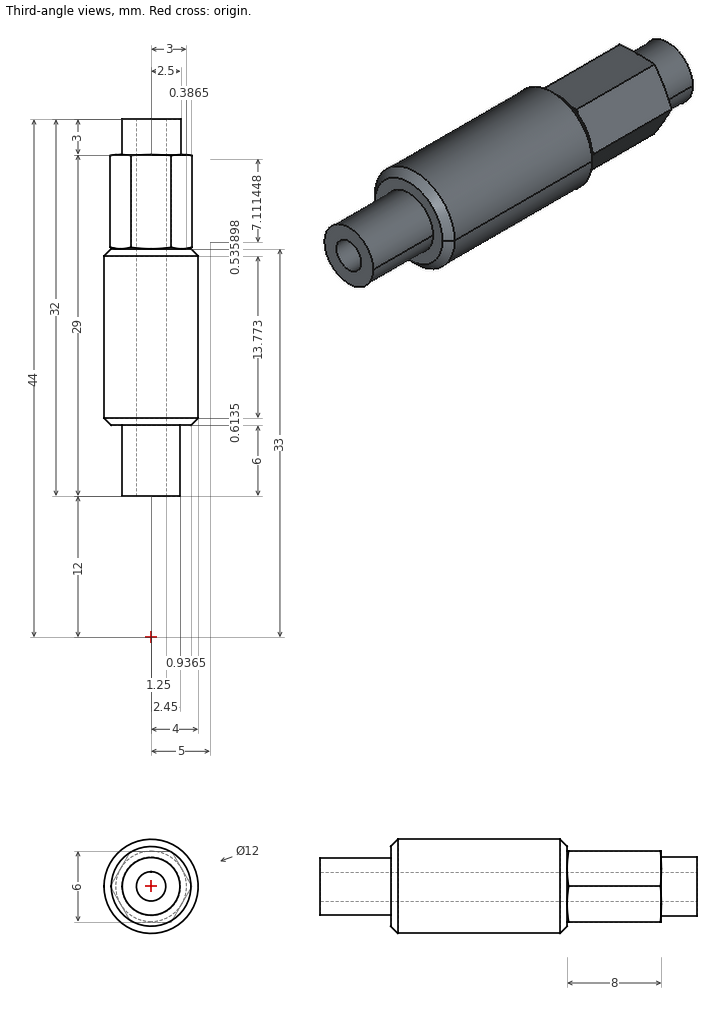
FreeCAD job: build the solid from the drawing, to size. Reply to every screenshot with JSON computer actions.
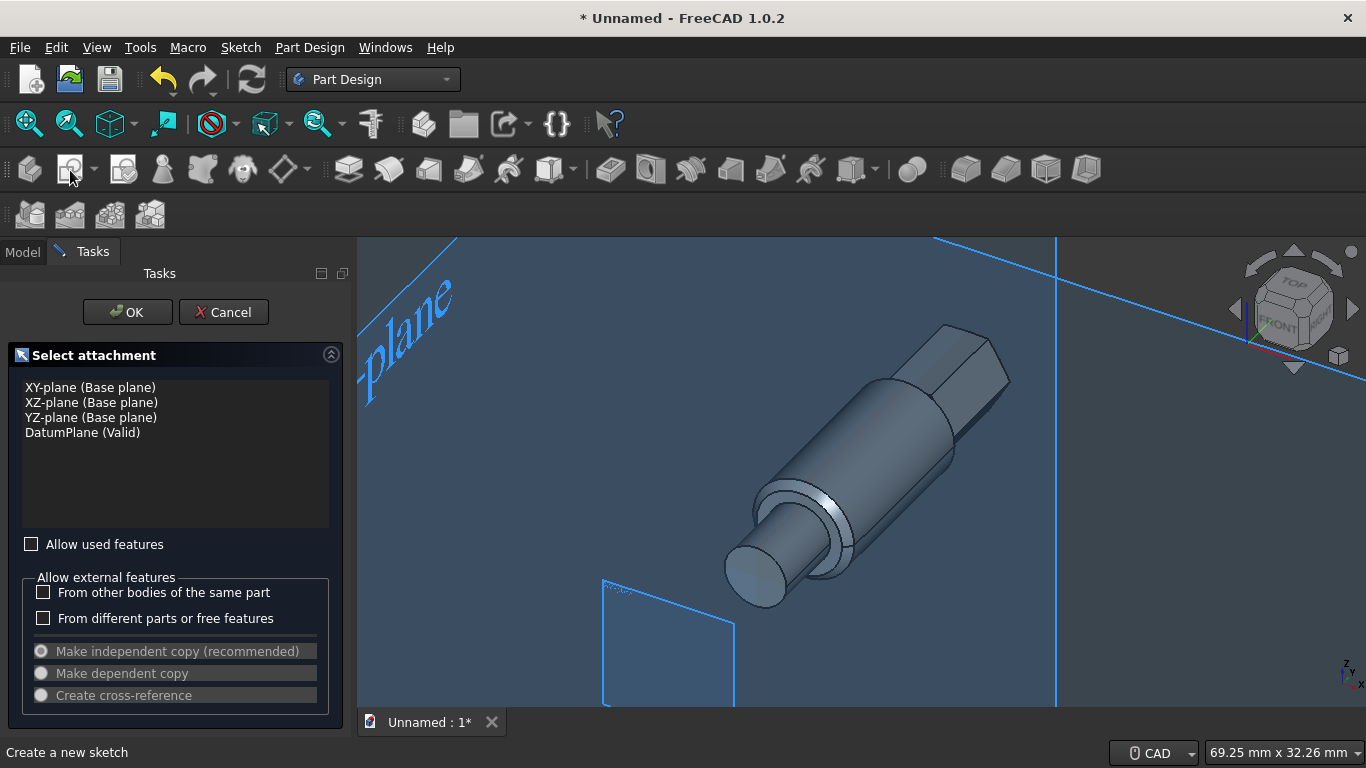
{"action": "left_click", "coordinate": [82, 388]}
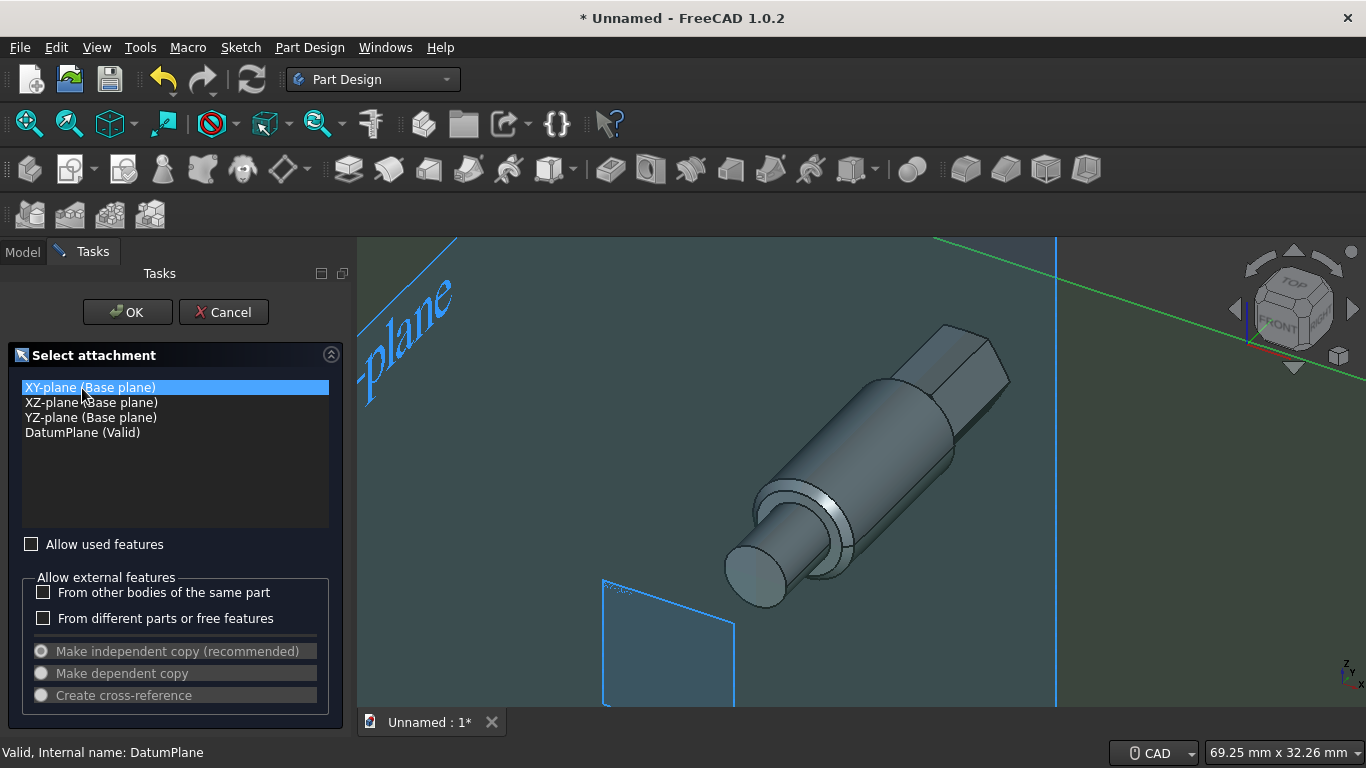
{"action": "left_click", "coordinate": [128, 312]}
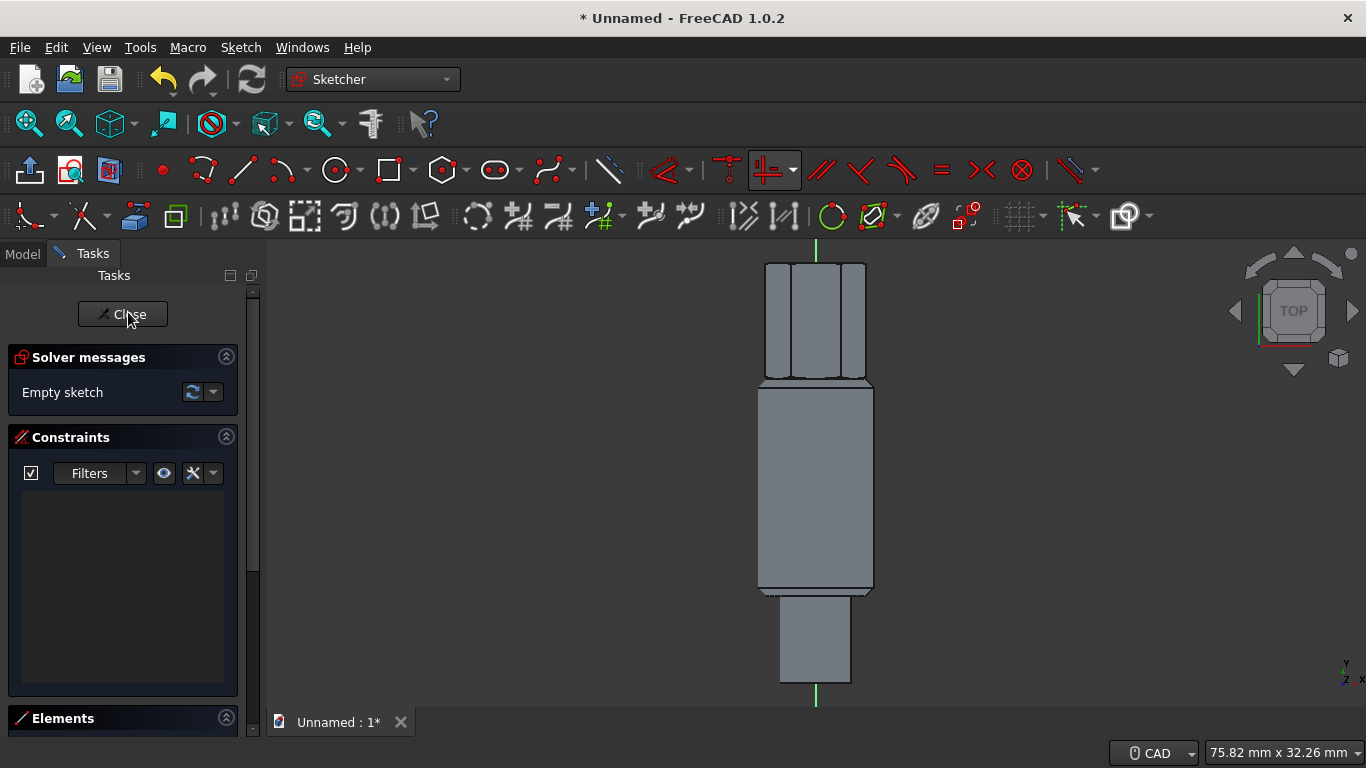
{"action": "left_click", "coordinate": [110, 170]}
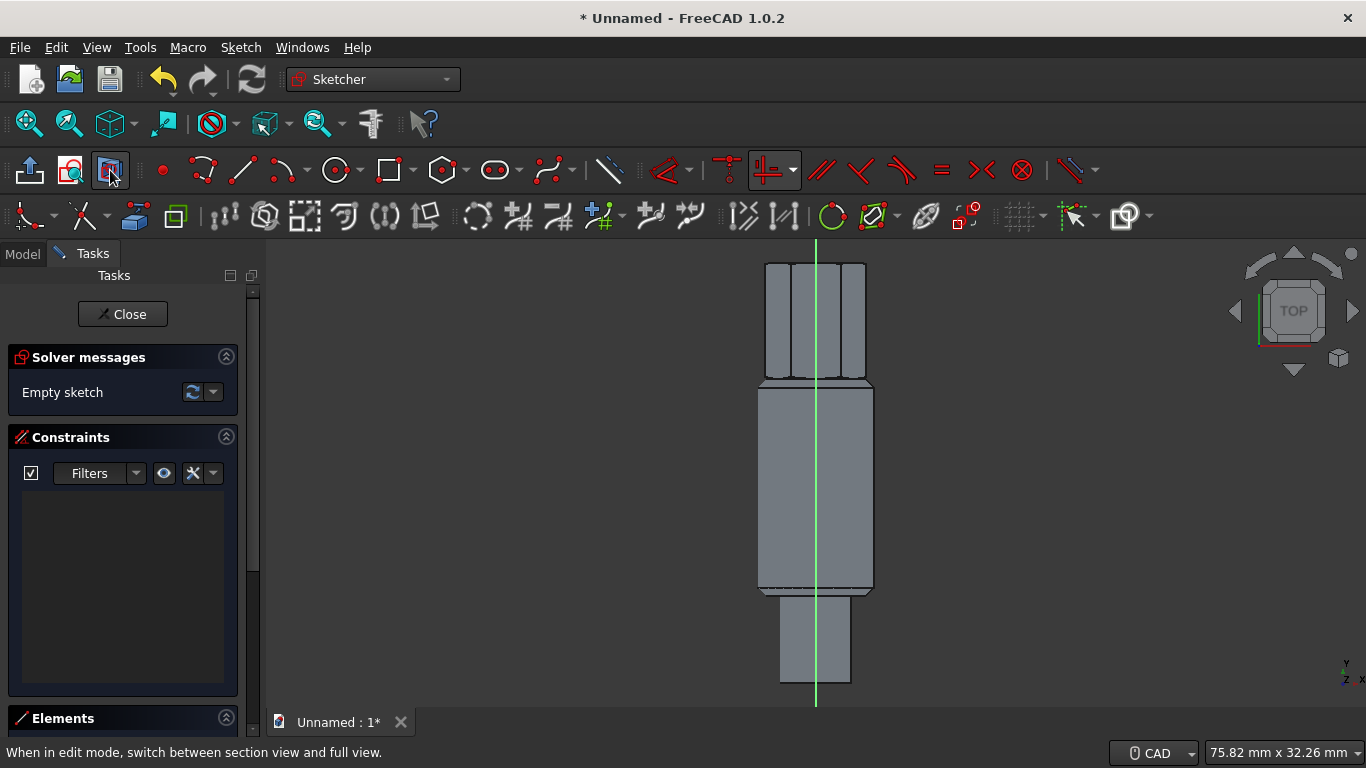
{"action": "scroll", "coordinate": [748, 473], "scroll_direction": "down", "scroll_amount": 5}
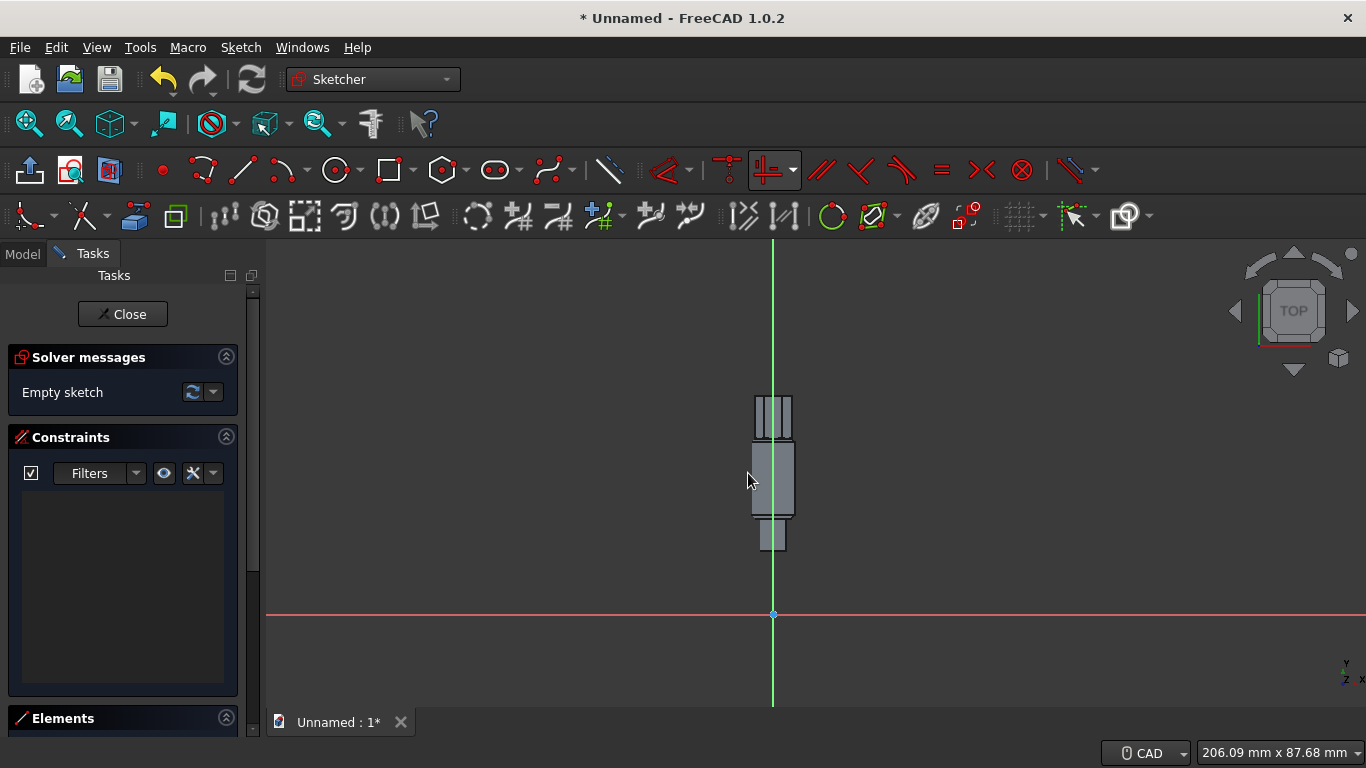
{"action": "scroll", "coordinate": [782, 382], "scroll_direction": "up", "scroll_amount": 14}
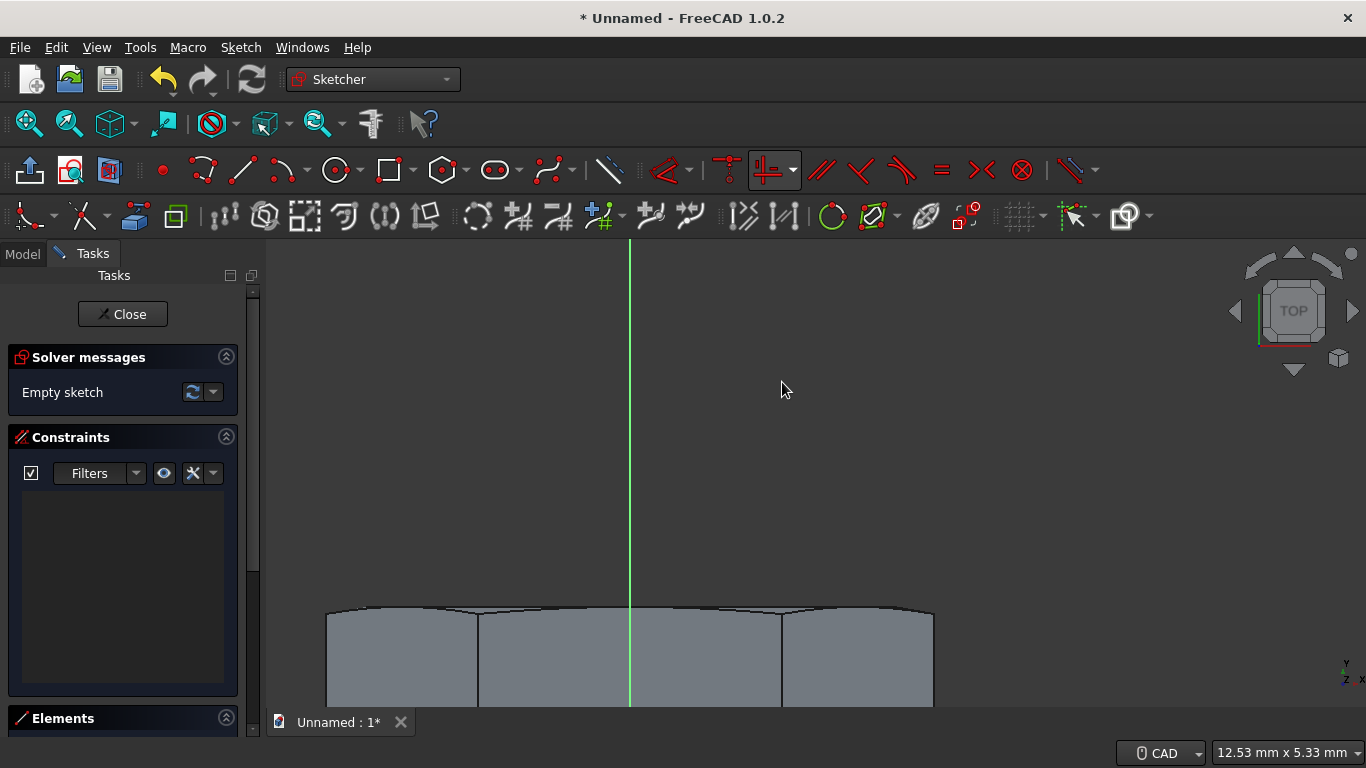
{"action": "left_click", "coordinate": [390, 170]}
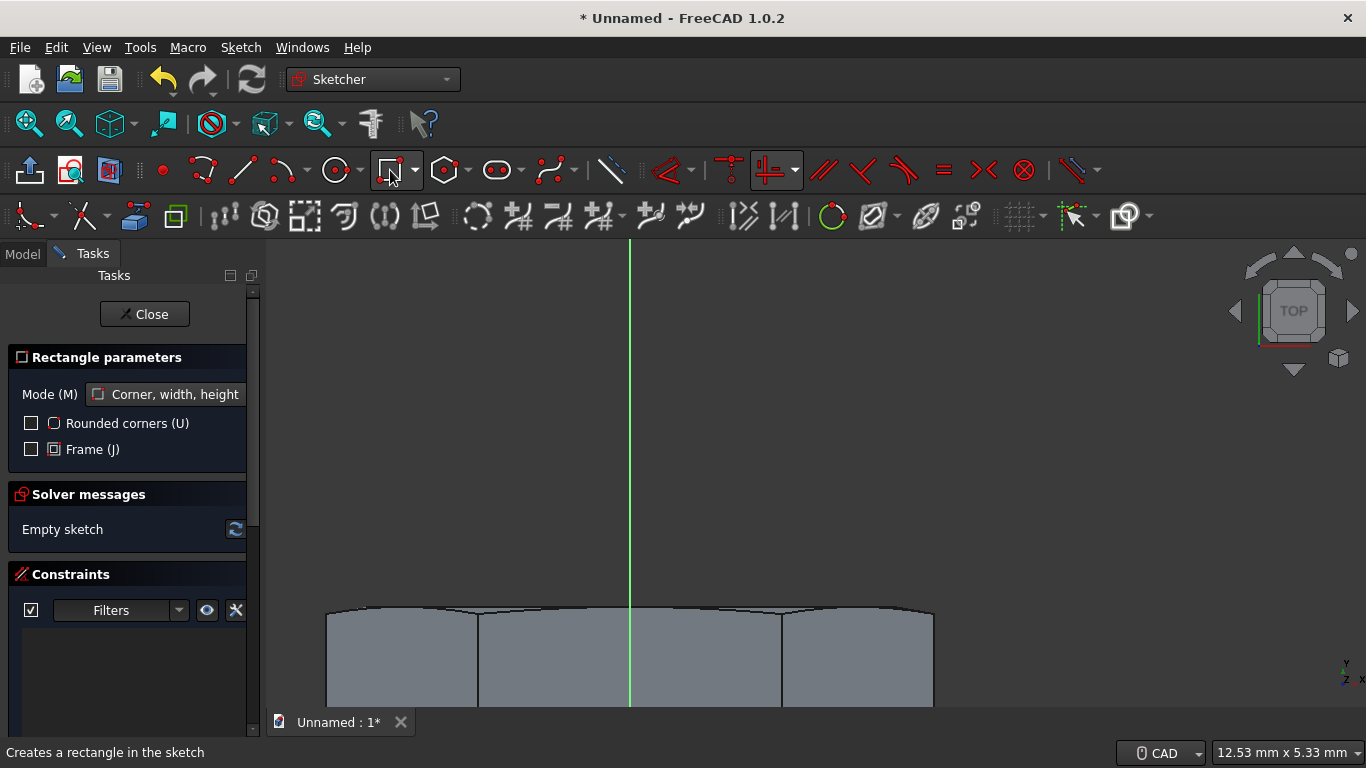
{"action": "left_click", "coordinate": [630, 344]}
{"action": "left_click", "coordinate": [849, 607]}
{"action": "key", "text": "Escape"}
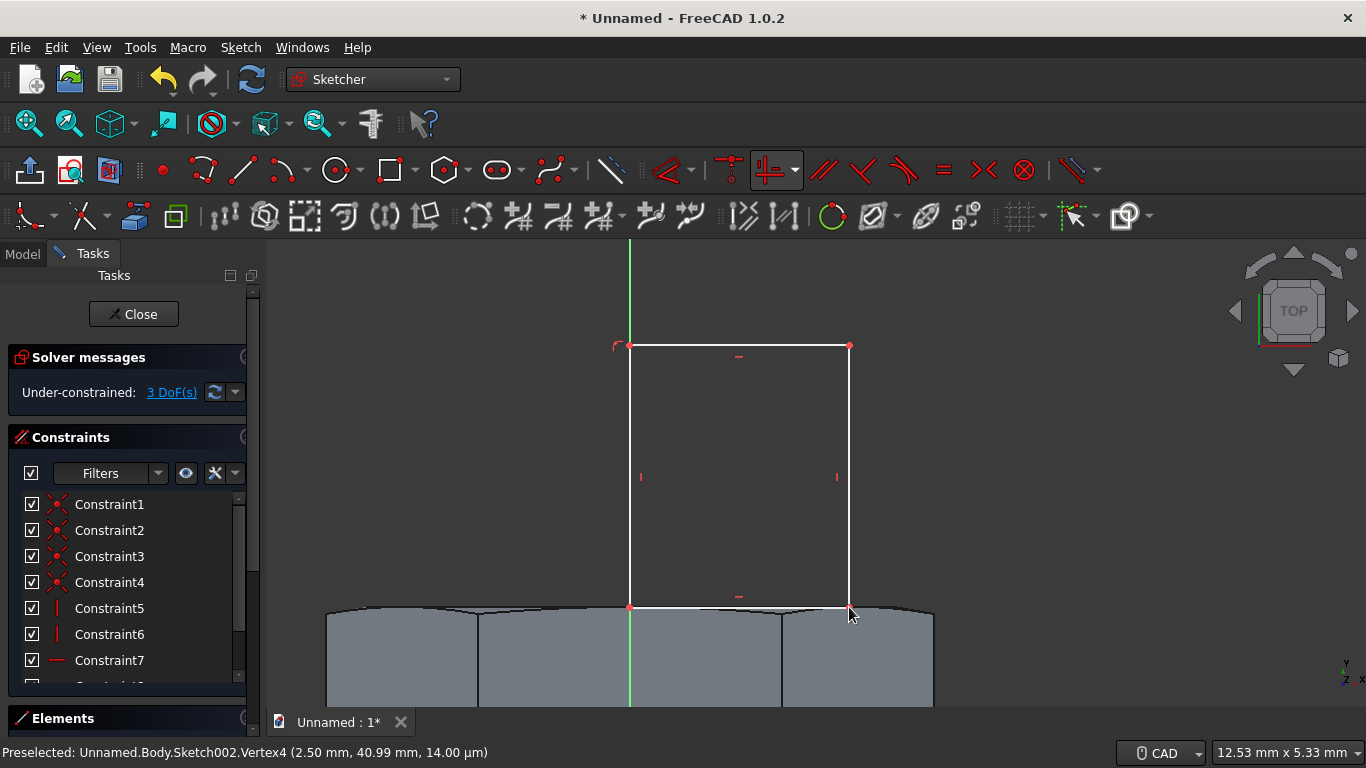
{"action": "left_click", "coordinate": [666, 170]}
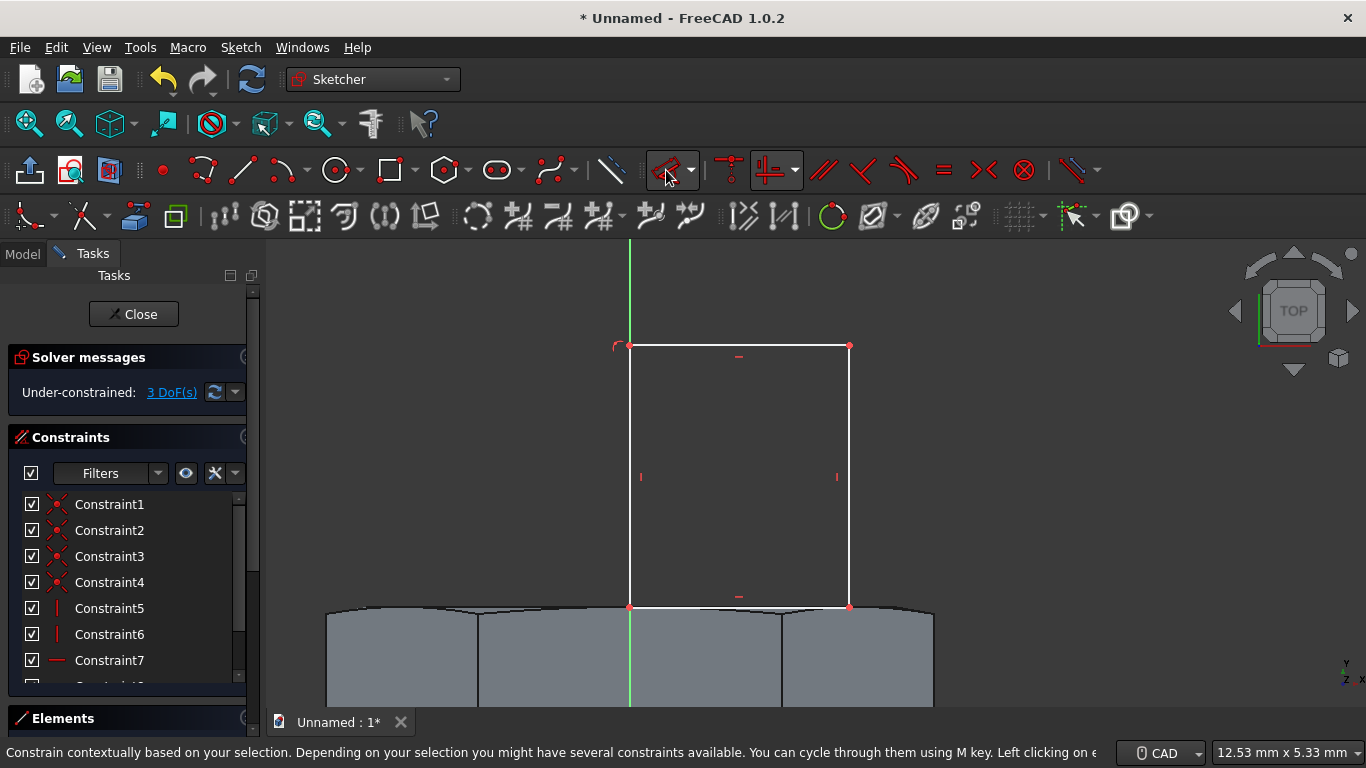
{"action": "left_click", "coordinate": [630, 424]}
{"action": "left_click", "coordinate": [596, 477]}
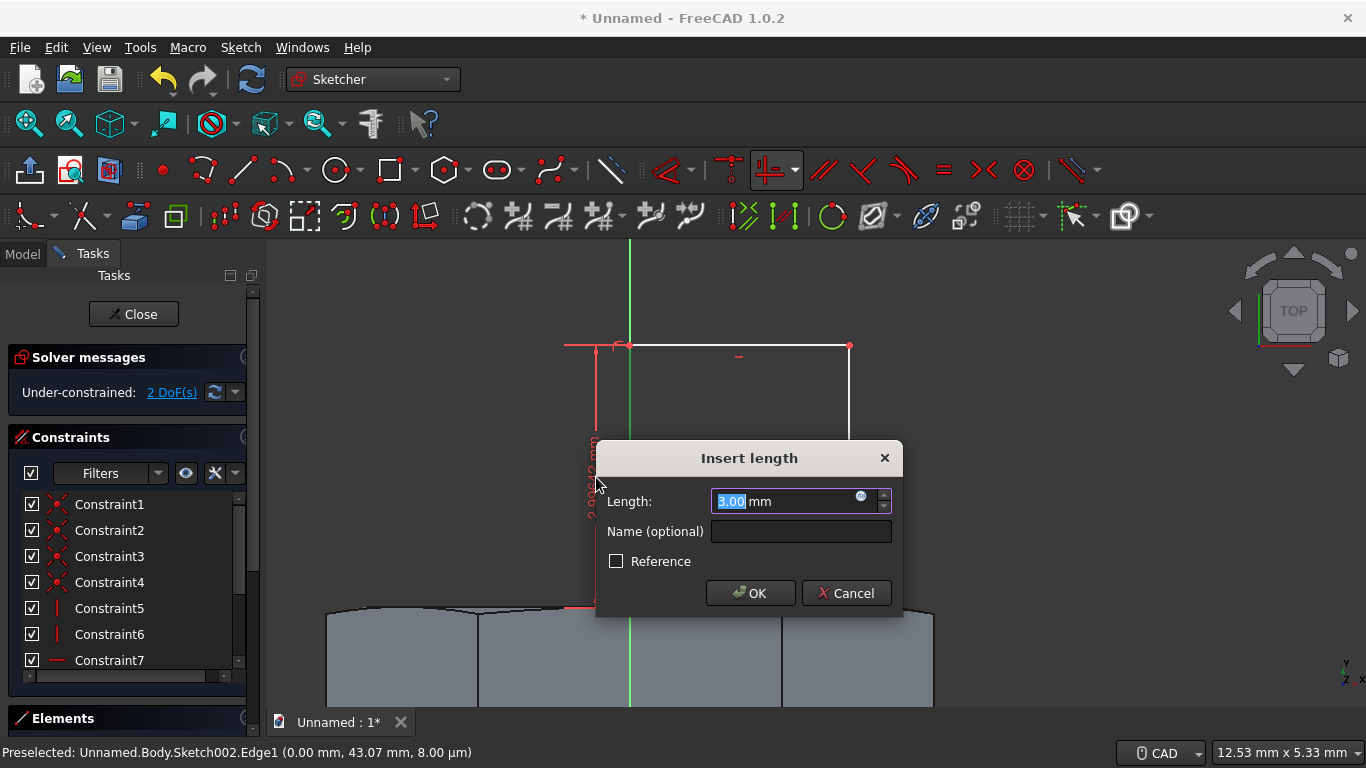
{"action": "type", "text": "3"}
{"action": "key", "text": "Return"}